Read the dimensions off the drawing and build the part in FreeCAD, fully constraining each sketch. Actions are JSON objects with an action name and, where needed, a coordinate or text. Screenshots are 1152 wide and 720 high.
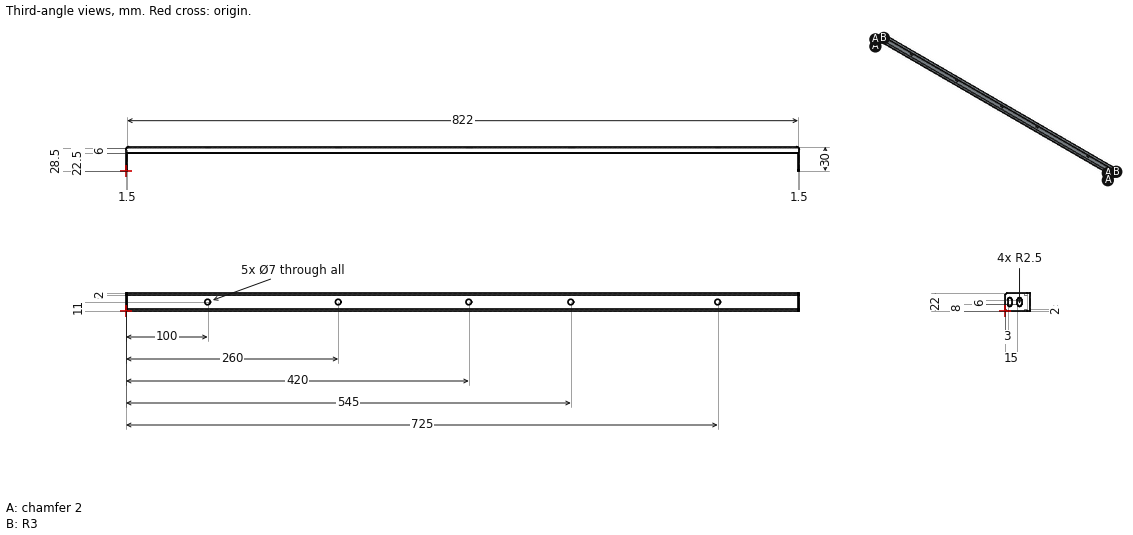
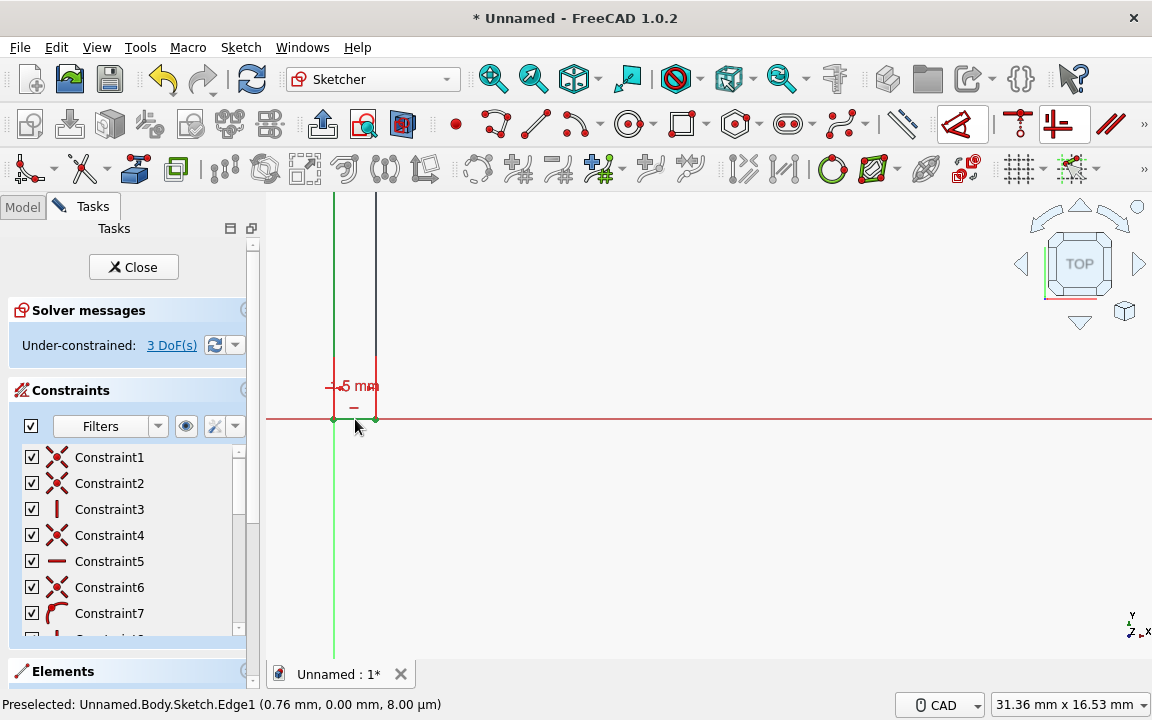
{"action": "scroll", "coordinate": [322, 438], "scroll_direction": "down", "scroll_amount": 18}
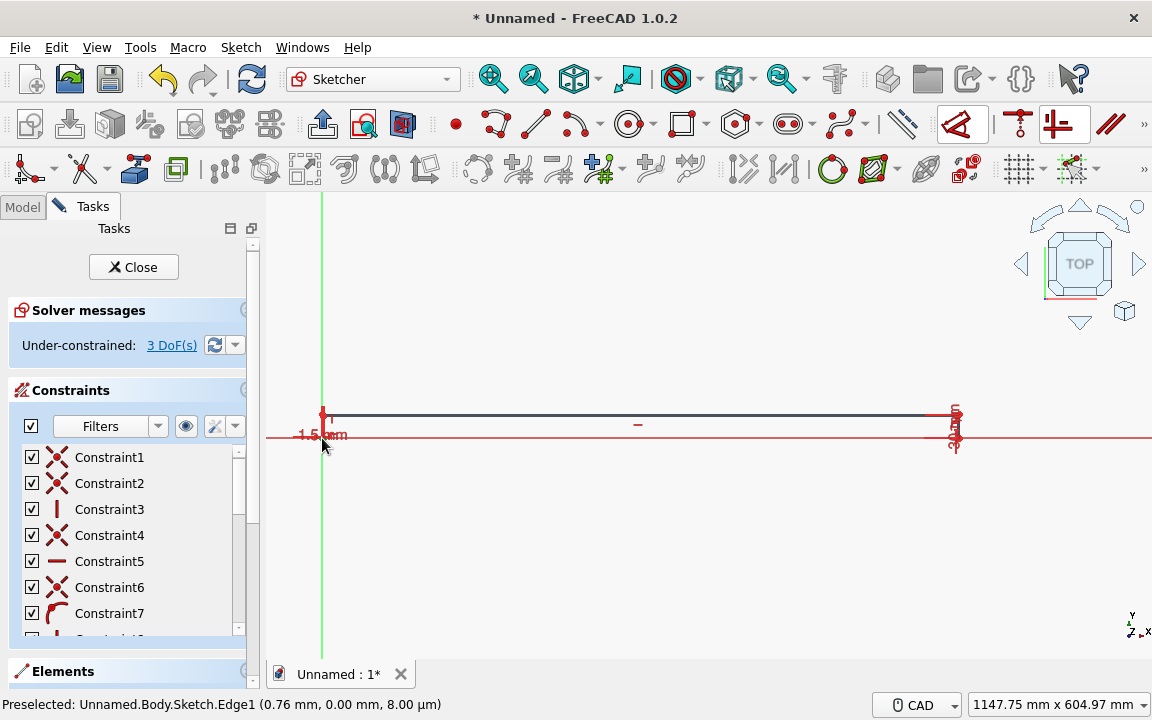
{"action": "scroll", "coordinate": [514, 416], "scroll_direction": "up", "scroll_amount": 13}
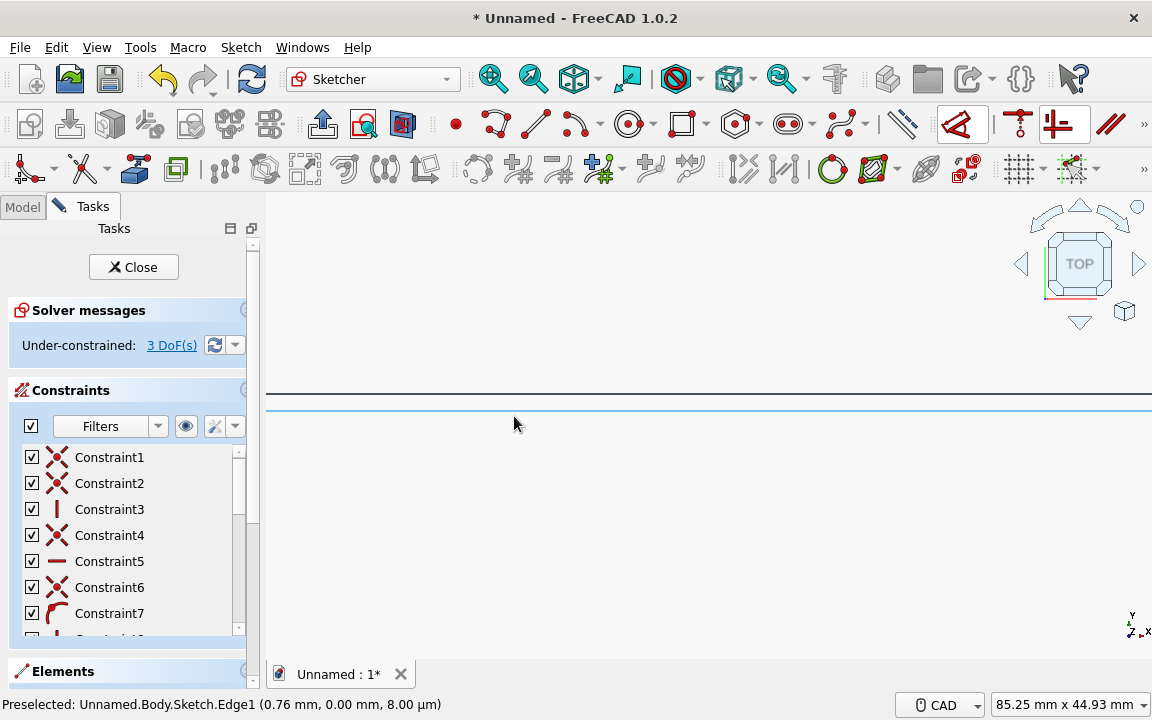
{"action": "left_click", "coordinate": [509, 411]}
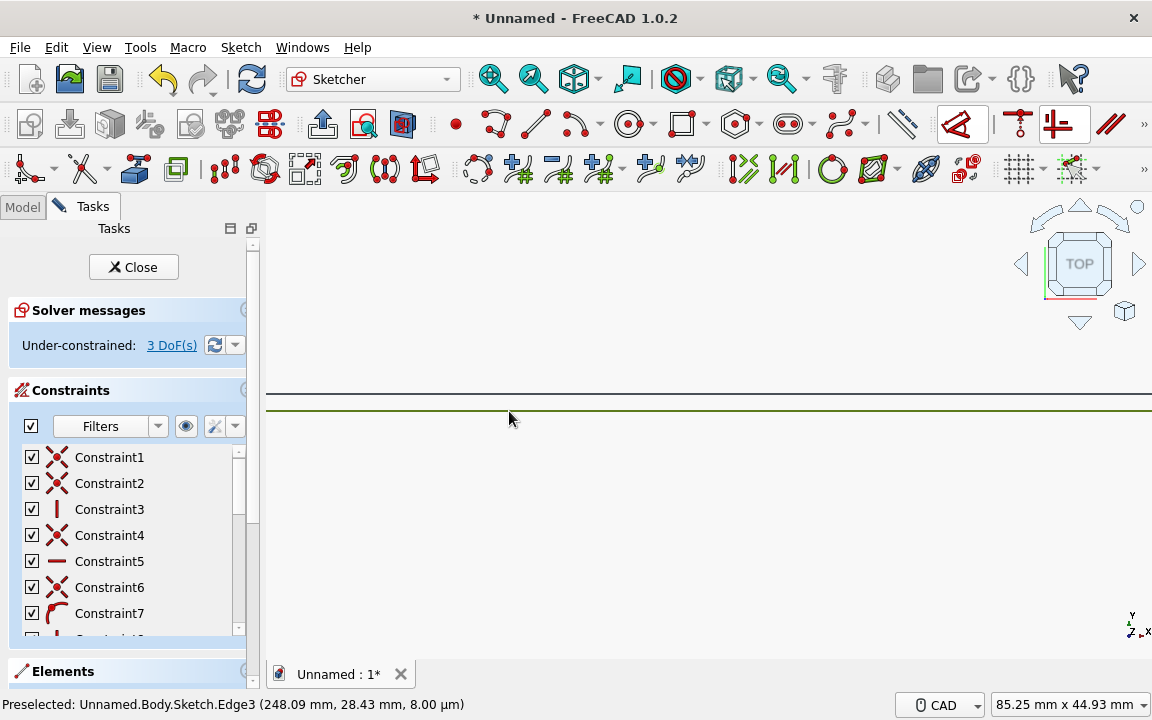
{"action": "left_click", "coordinate": [982, 124]}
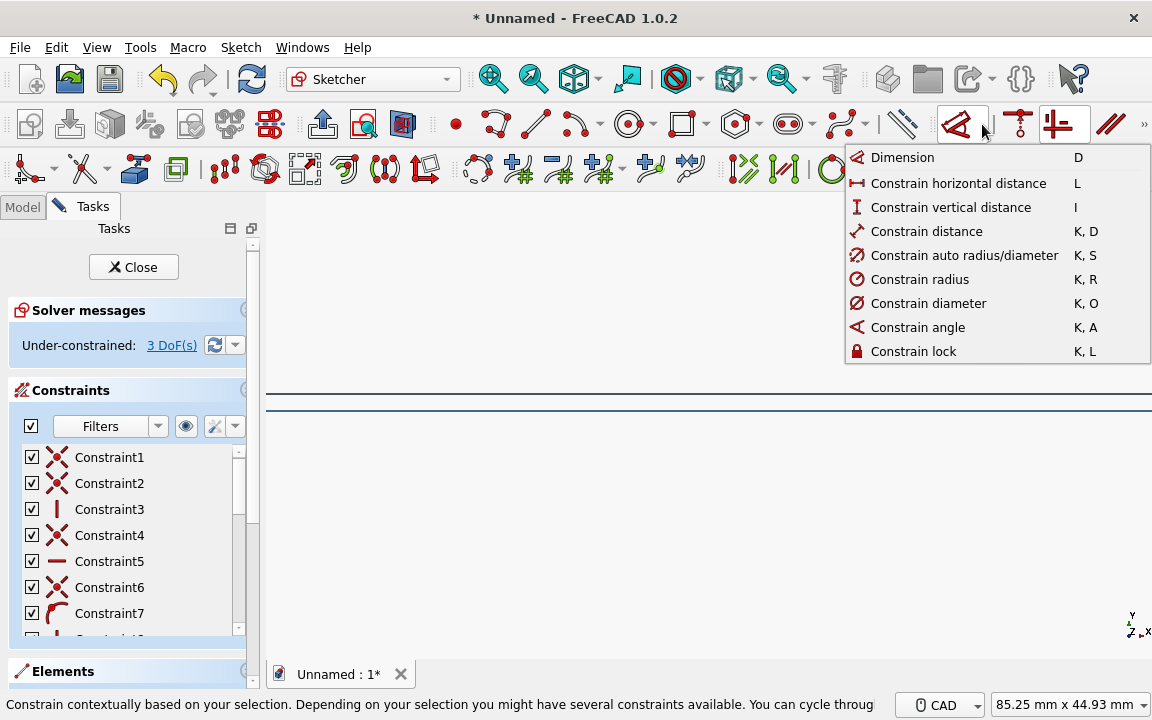
{"action": "left_click", "coordinate": [998, 183]}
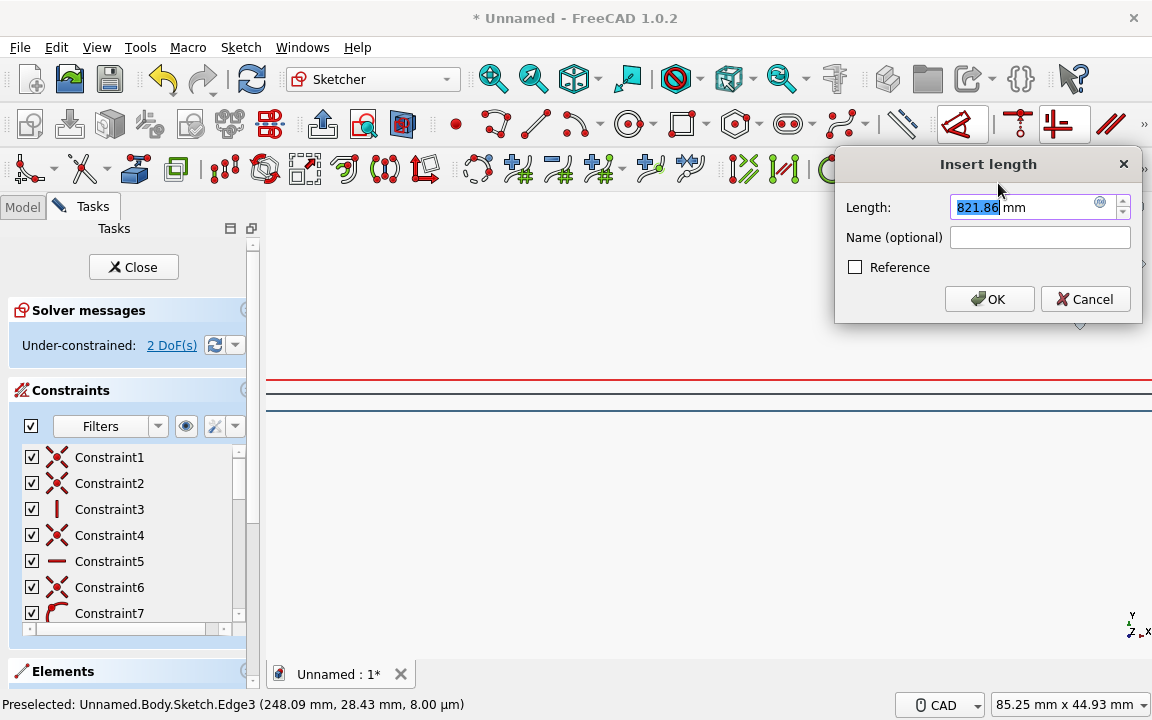
{"action": "type", "text": "822"}
{"action": "key", "text": "Return"}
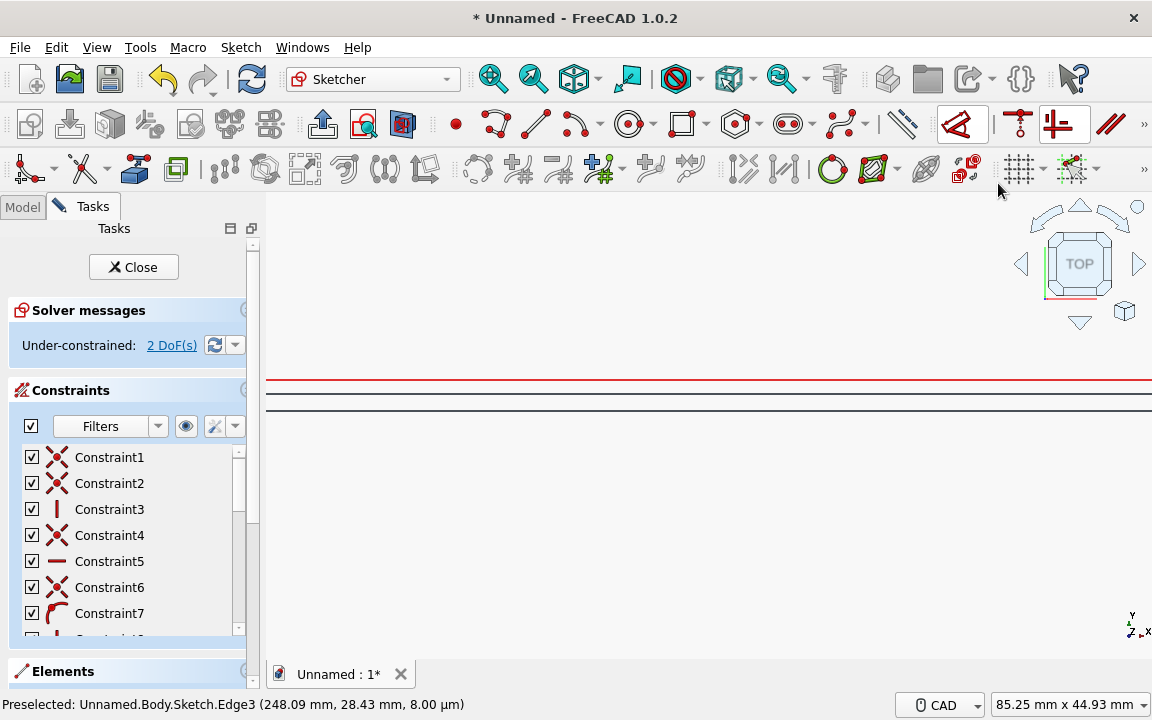
{"action": "scroll", "coordinate": [538, 417], "scroll_direction": "down", "scroll_amount": 14}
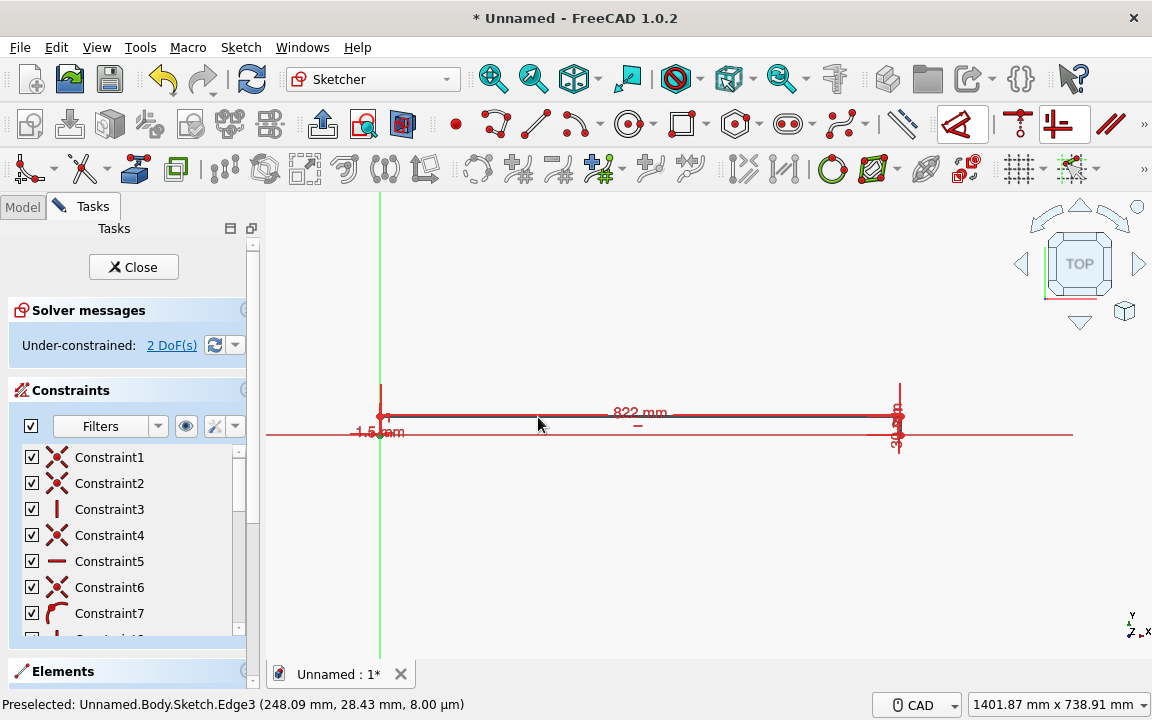
{"action": "scroll", "coordinate": [901, 435], "scroll_direction": "up", "scroll_amount": 19}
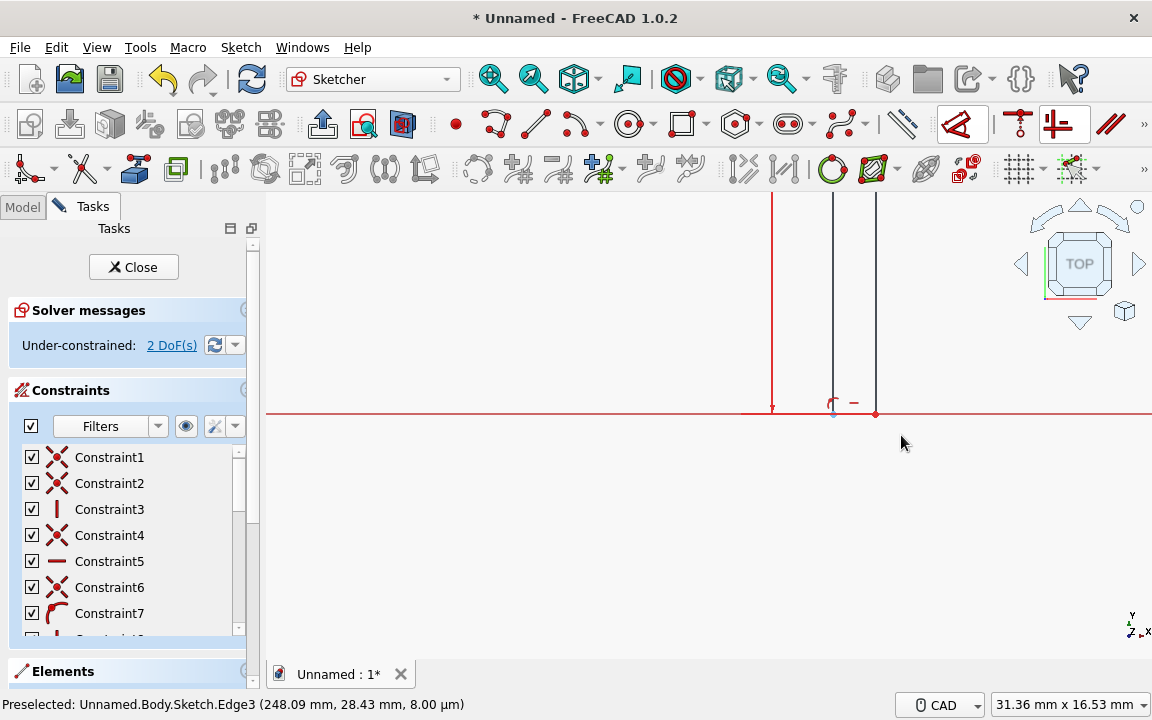
{"action": "left_click", "coordinate": [855, 414]}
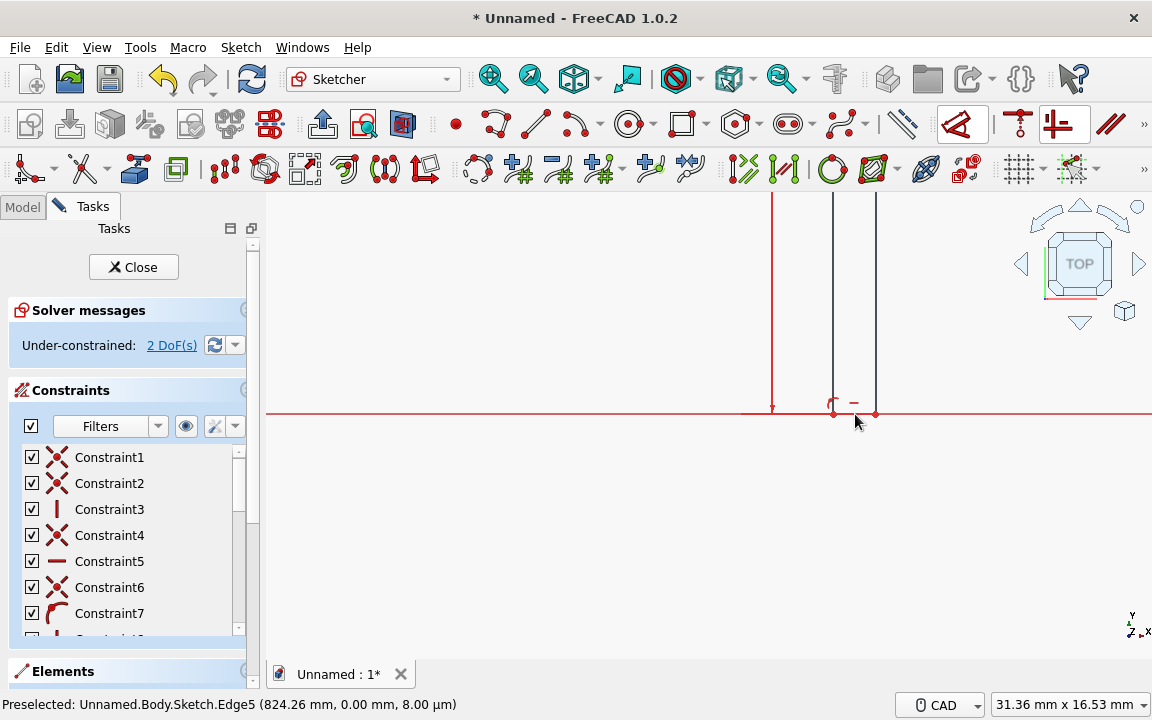
{"action": "key", "text": "l"}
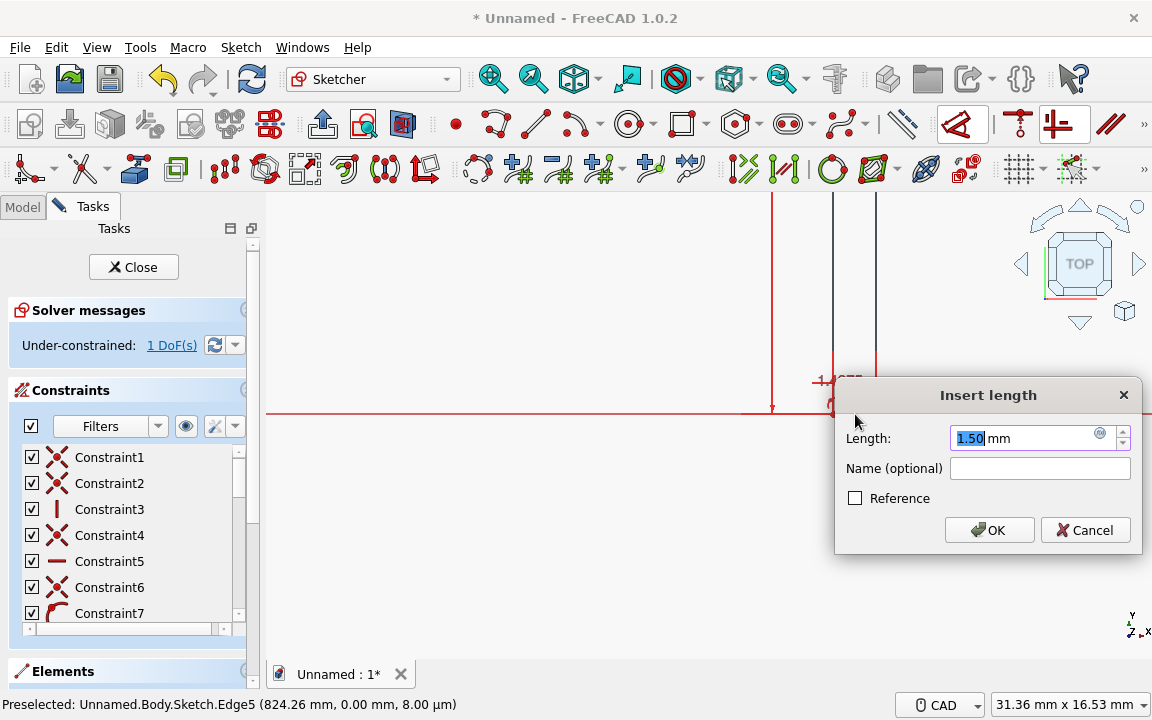
{"action": "type", "text": "1.5"}
{"action": "key", "text": "Return"}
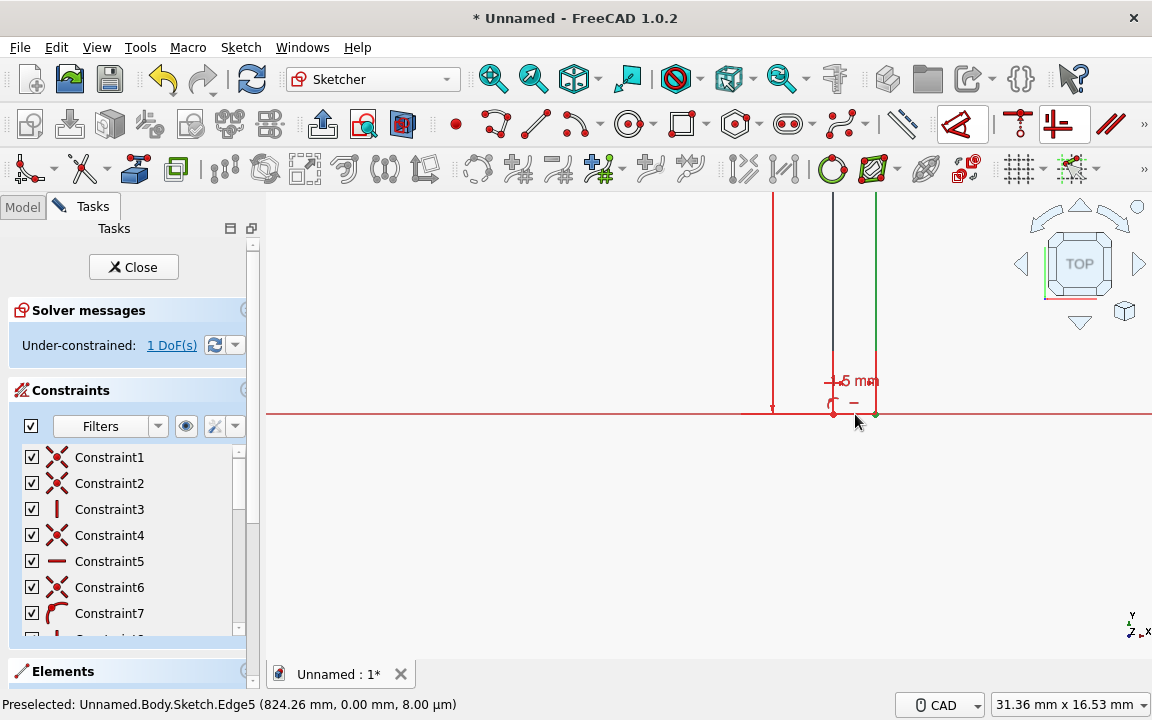
{"action": "scroll", "coordinate": [961, 438], "scroll_direction": "down", "scroll_amount": 18}